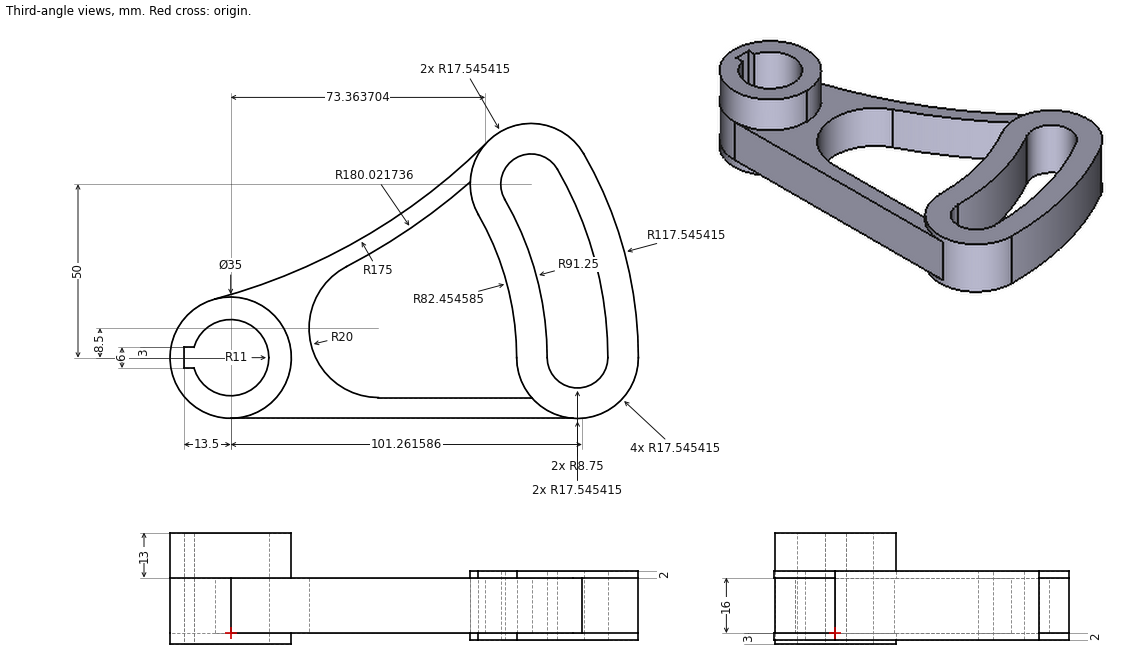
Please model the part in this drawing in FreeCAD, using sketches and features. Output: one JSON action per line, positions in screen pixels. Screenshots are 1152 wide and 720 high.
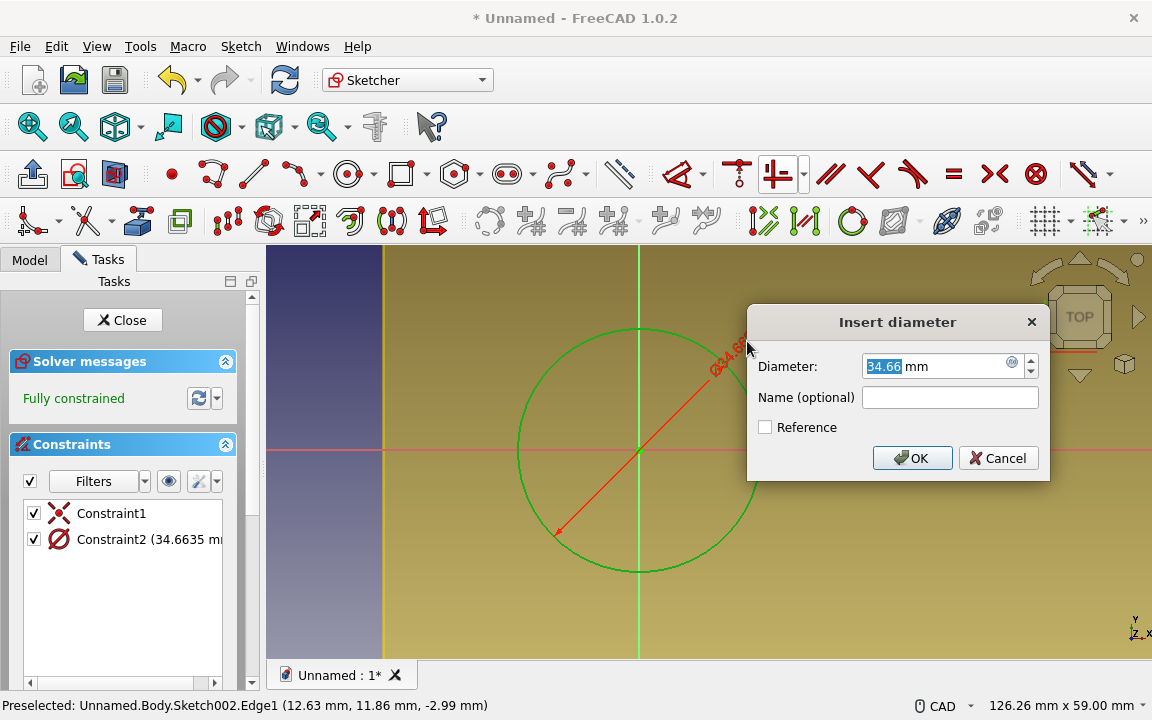
{"action": "type", "text": "35"}
{"action": "key", "text": "Return"}
{"action": "key", "text": "Escape"}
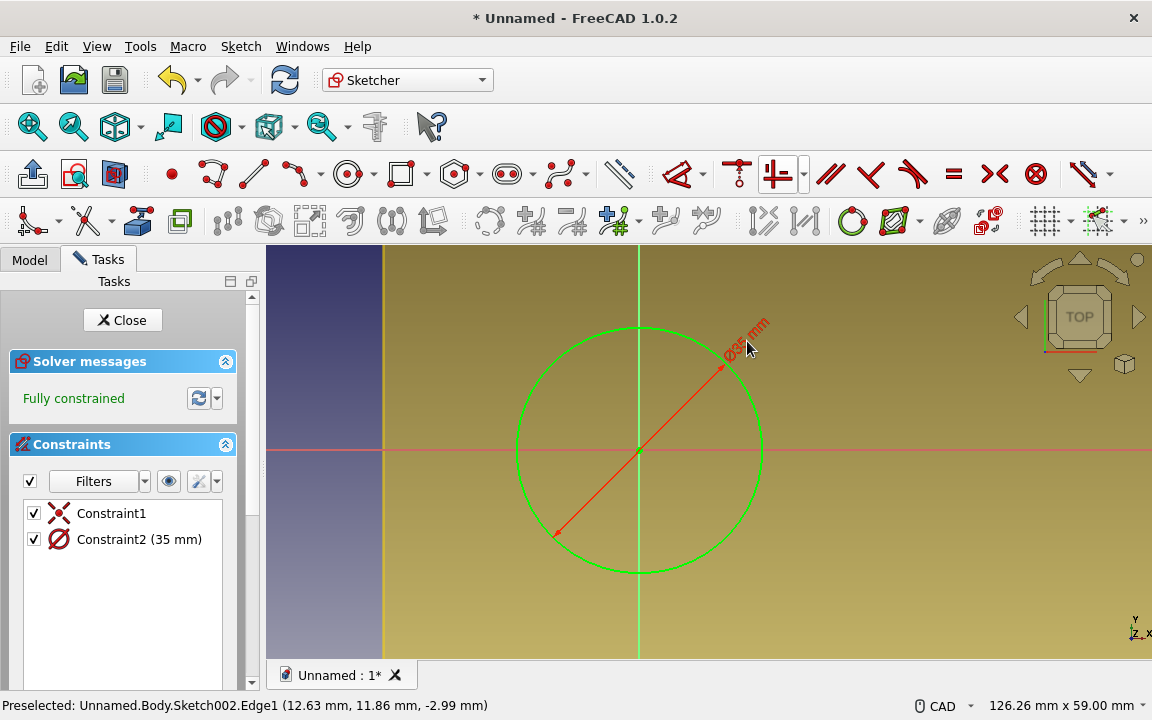
{"action": "left_click", "coordinate": [123, 320]}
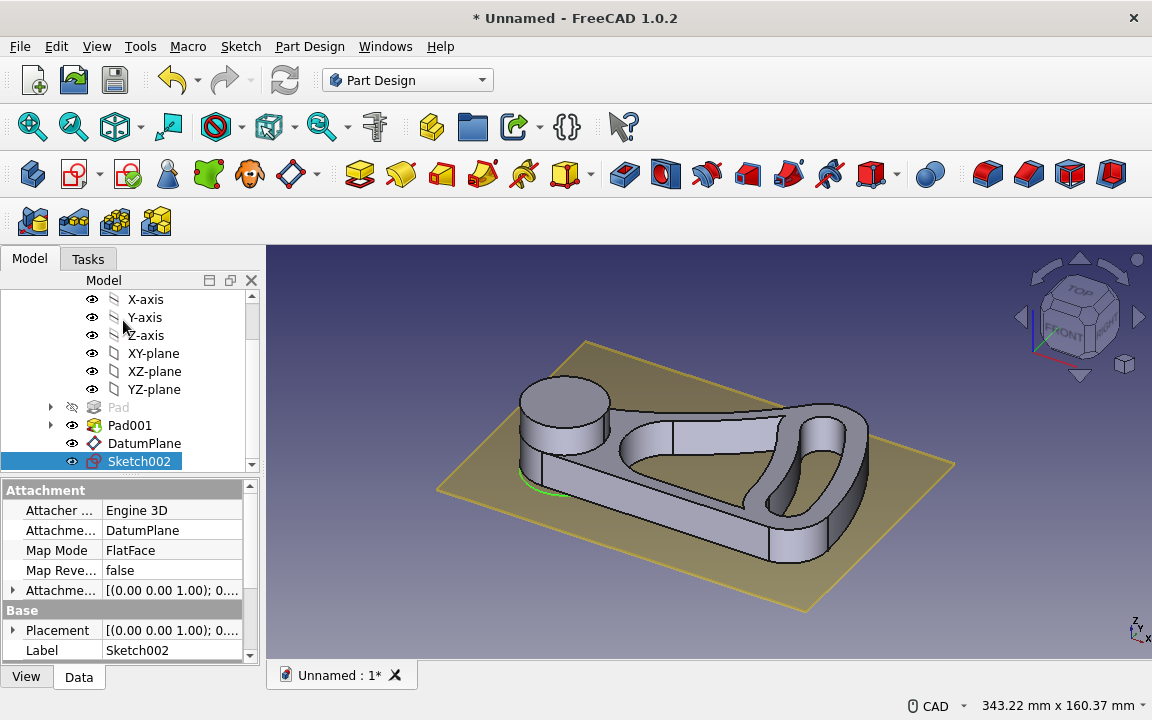
{"action": "left_click", "coordinate": [360, 174]}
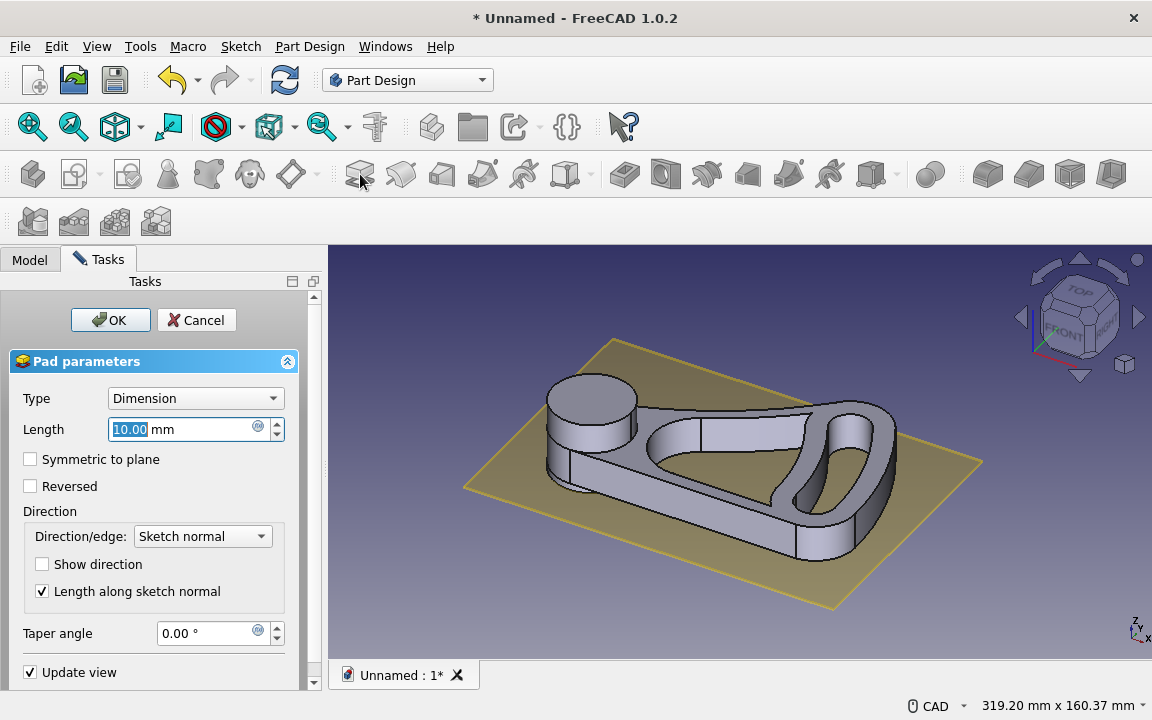
{"action": "type", "text": "3"}
{"action": "key", "text": "Tab"}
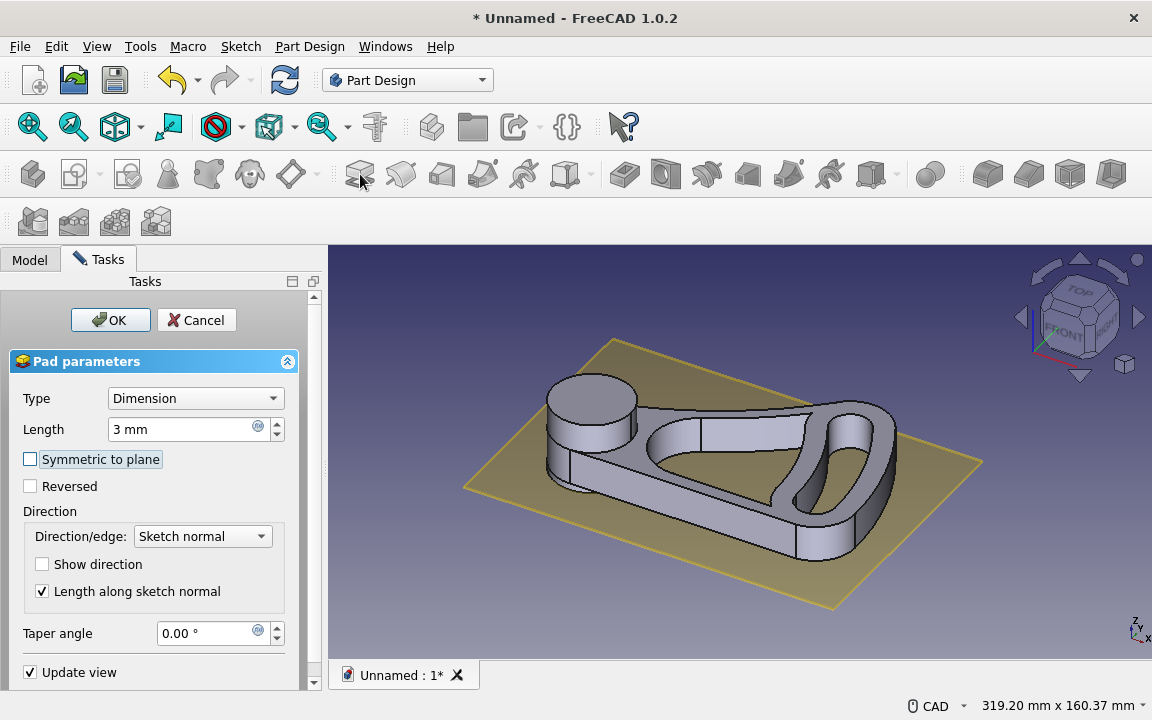
{"action": "left_click", "coordinate": [111, 320]}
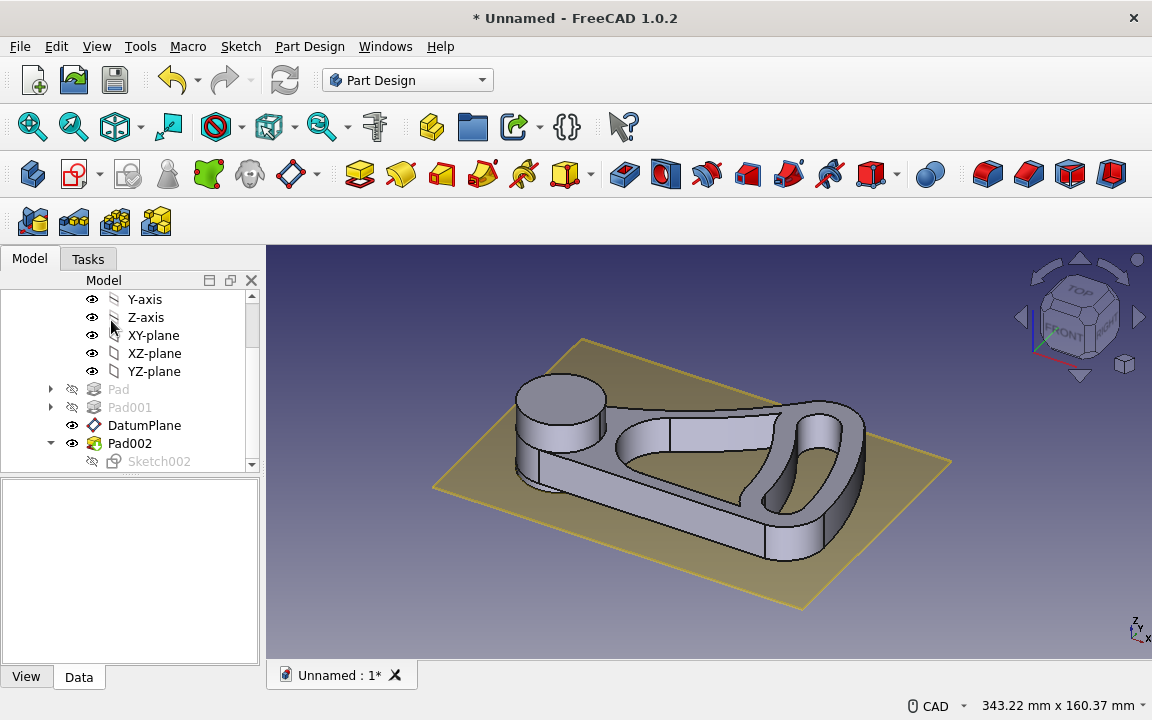
{"action": "left_click", "coordinate": [117, 425]}
{"action": "key", "text": "space"}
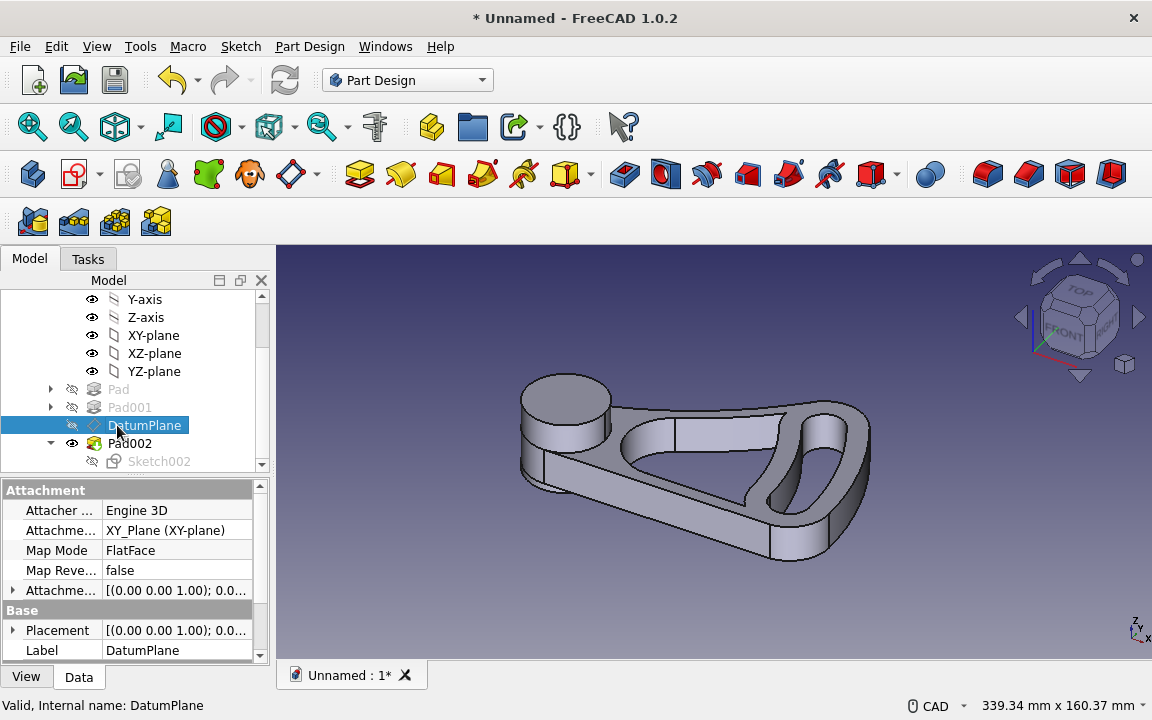
{"action": "left_click", "coordinate": [566, 399]}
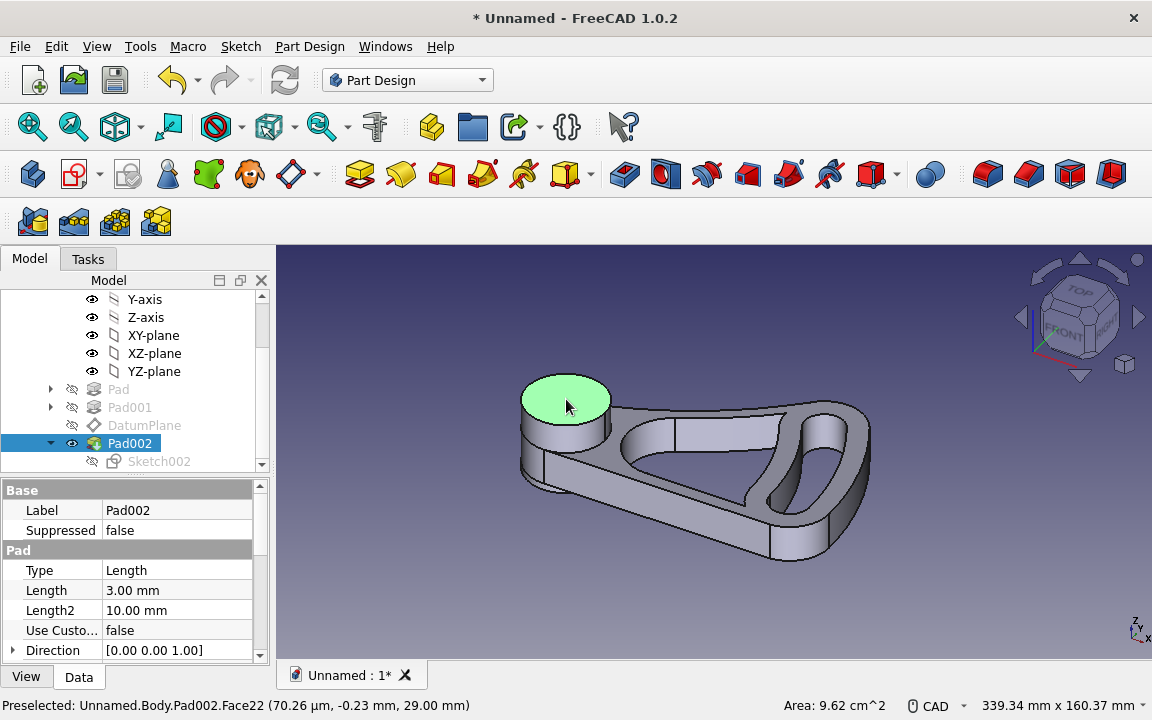
{"action": "left_click", "coordinate": [74, 174]}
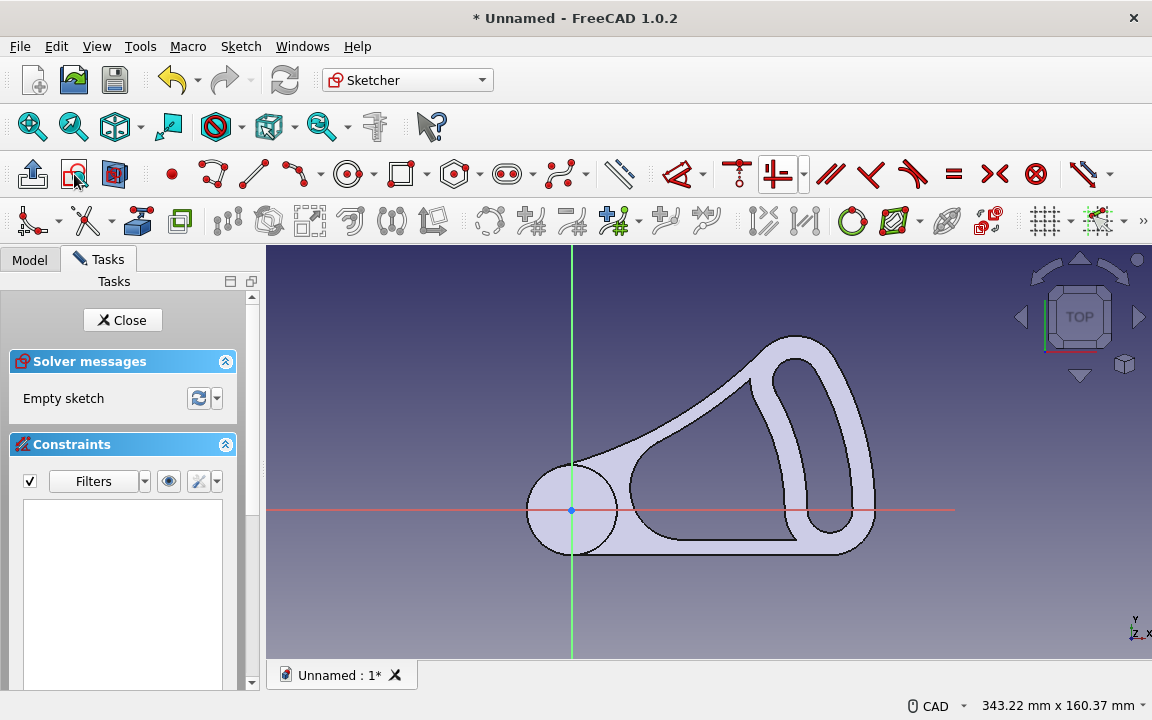
{"action": "scroll", "coordinate": [557, 519], "scroll_direction": "up", "scroll_amount": 10}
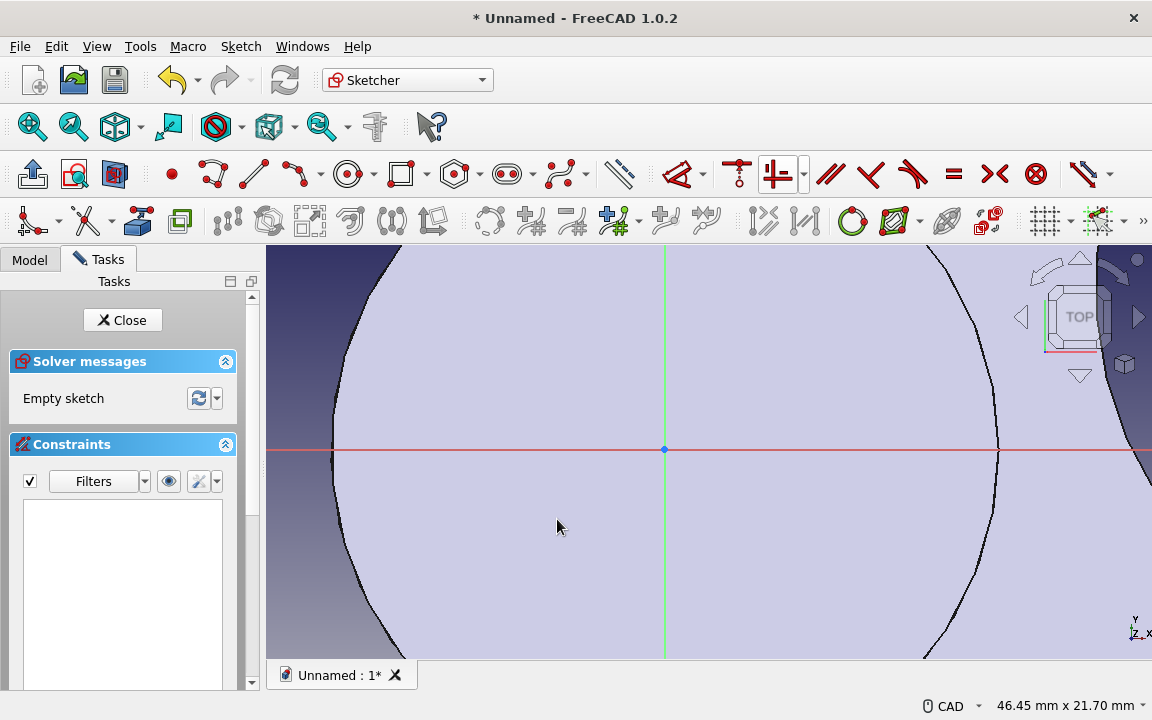
{"action": "left_click", "coordinate": [213, 174]}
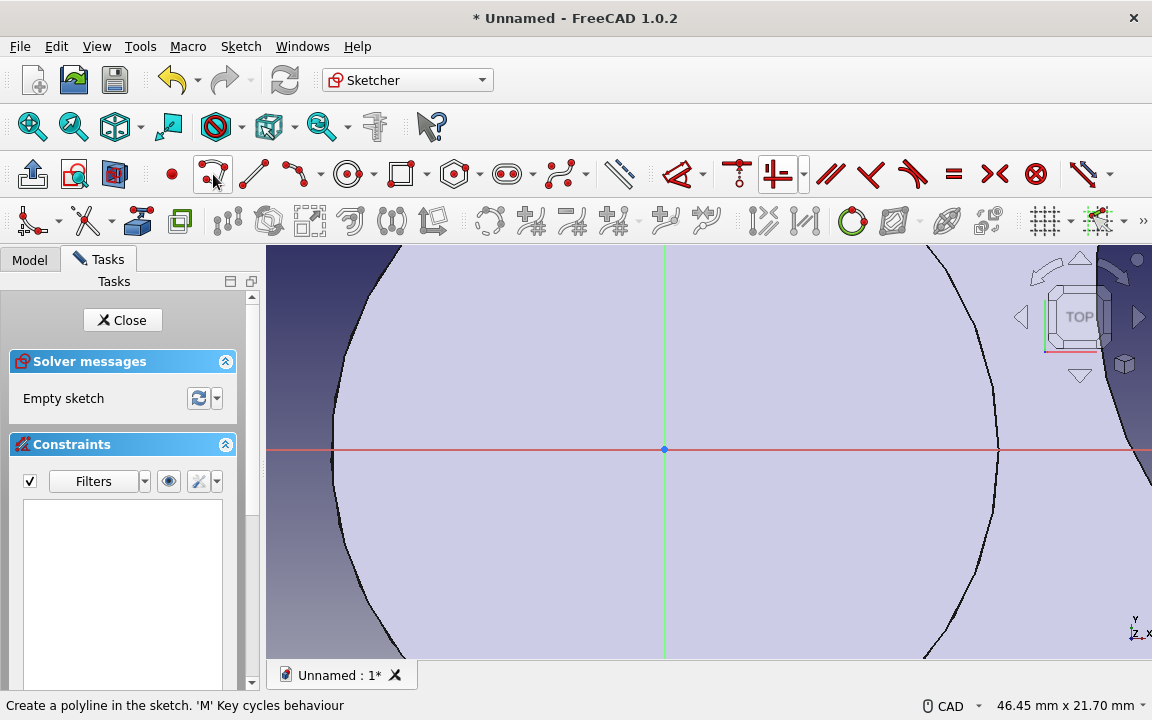
{"action": "left_click", "coordinate": [463, 393]}
{"action": "left_click", "coordinate": [407, 393]}
{"action": "left_click", "coordinate": [407, 507]}
{"action": "left_click", "coordinate": [463, 507]}
{"action": "right_click", "coordinate": [463, 507]}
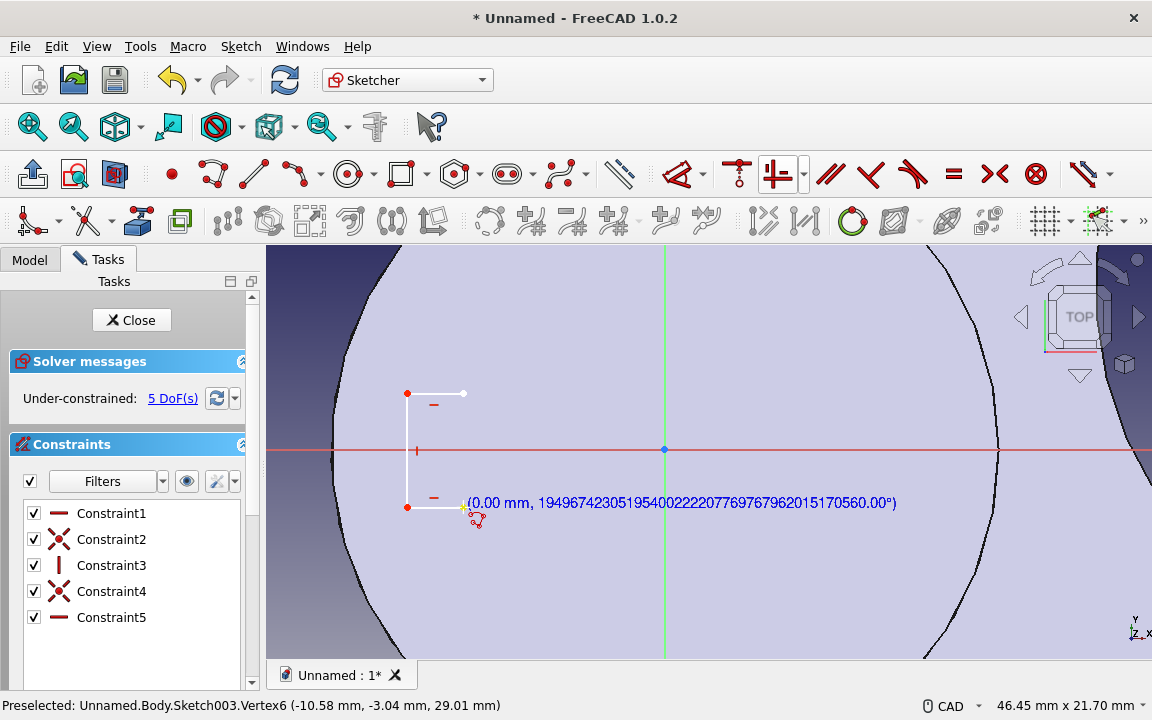
{"action": "left_click", "coordinate": [294, 174]}